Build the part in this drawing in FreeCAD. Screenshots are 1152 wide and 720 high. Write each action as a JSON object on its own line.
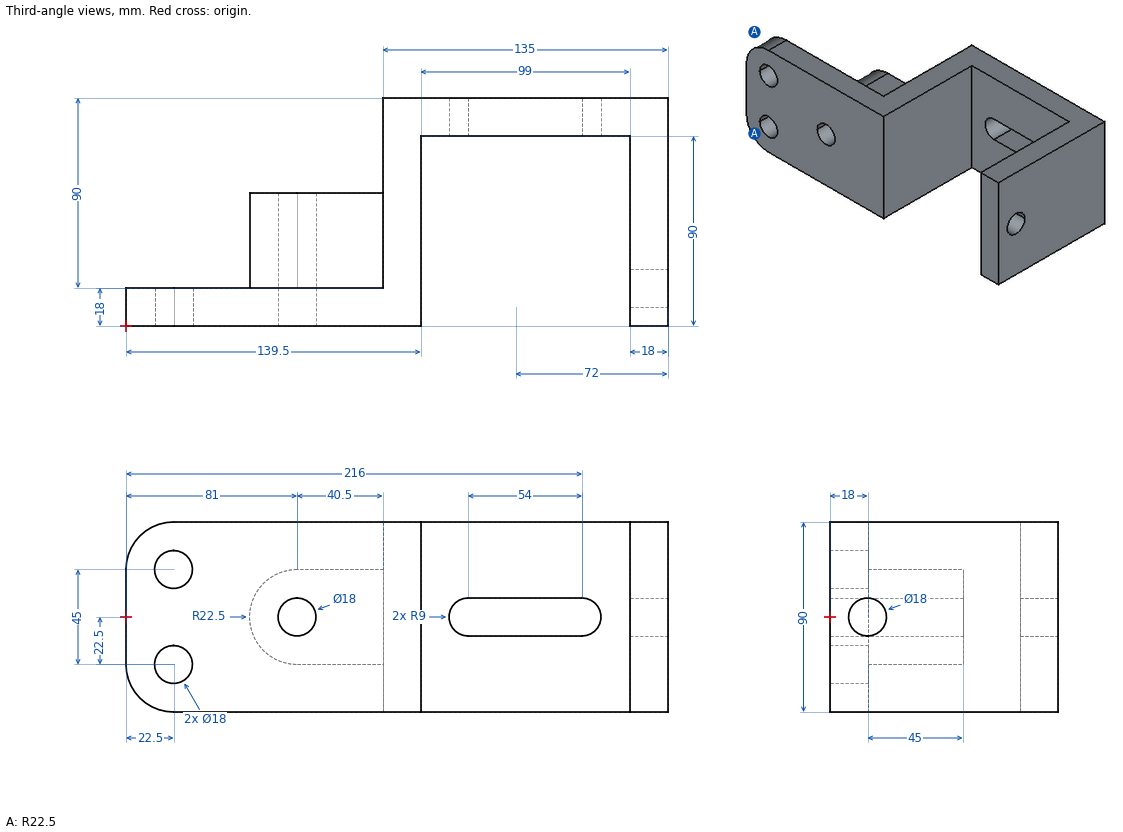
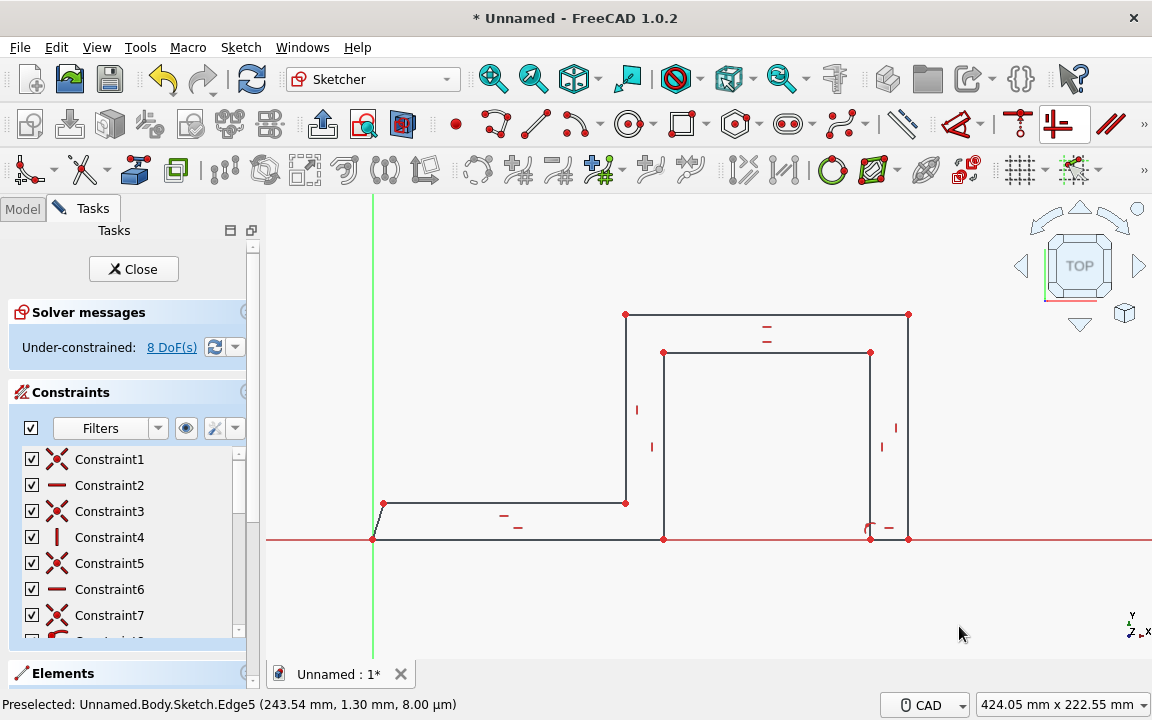
{"action": "scroll", "coordinate": [381, 514], "scroll_direction": "up", "scroll_amount": 3}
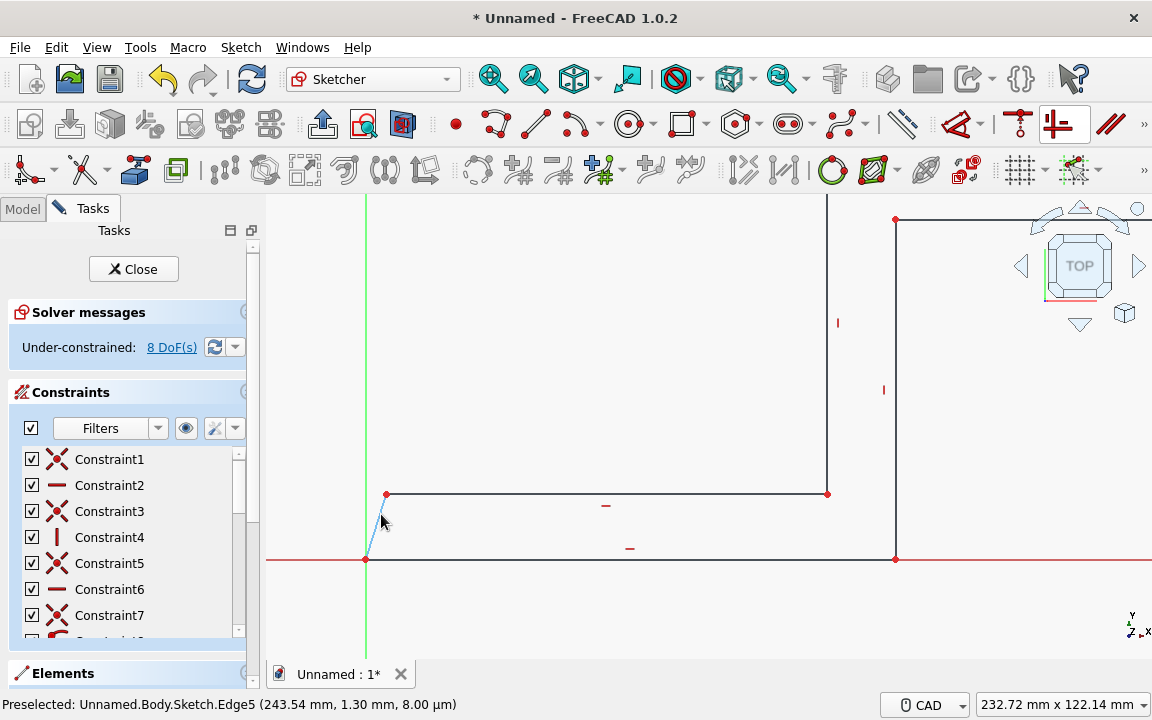
{"action": "left_click", "coordinate": [380, 514]}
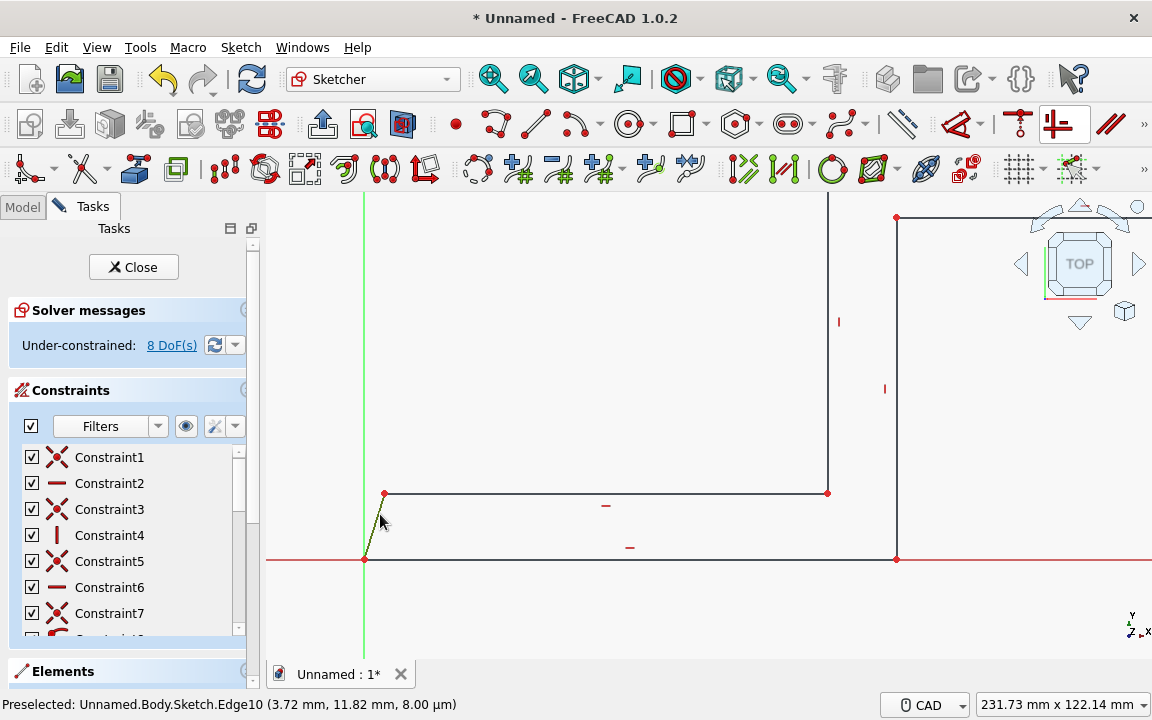
{"action": "left_click", "coordinate": [1084, 124]}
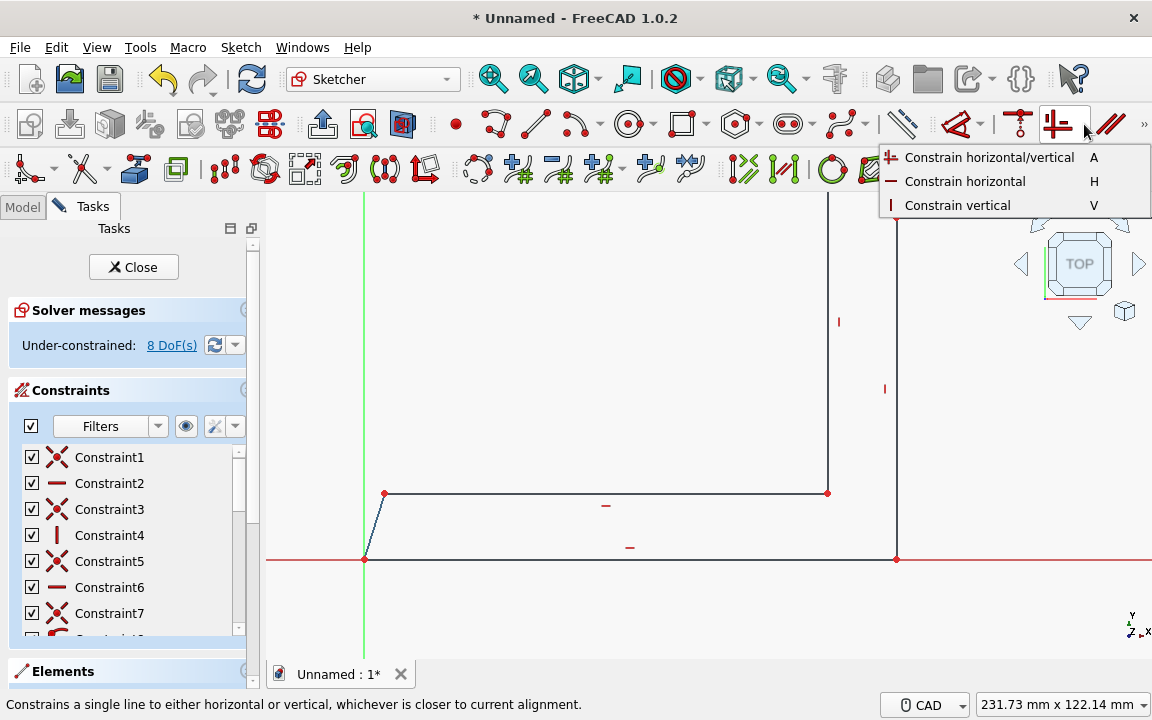
{"action": "left_click", "coordinate": [1015, 205]}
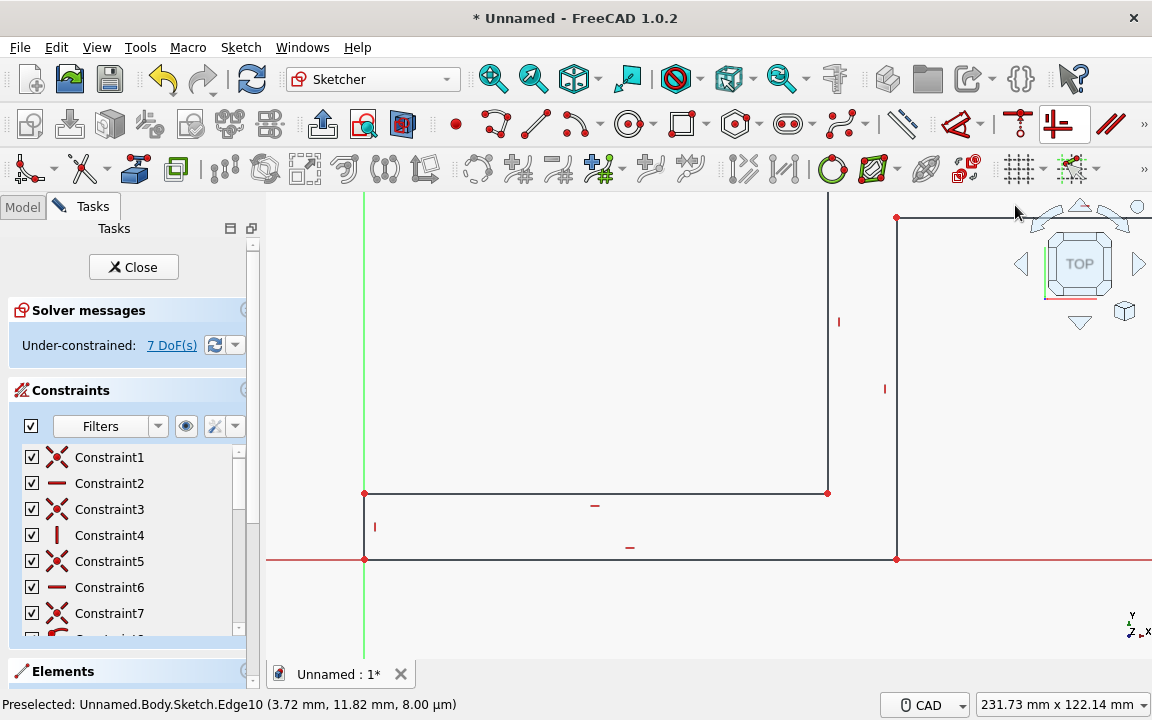
{"action": "left_click", "coordinate": [956, 124]}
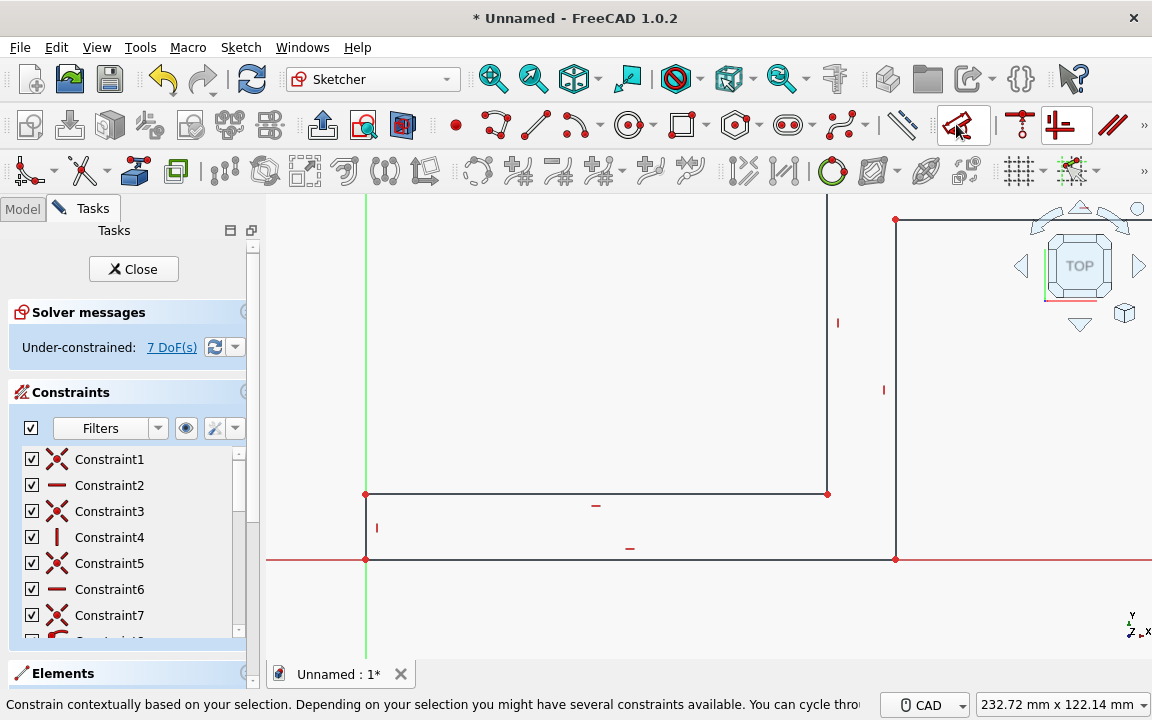
{"action": "left_click", "coordinate": [896, 458]}
{"action": "left_click", "coordinate": [930, 391]}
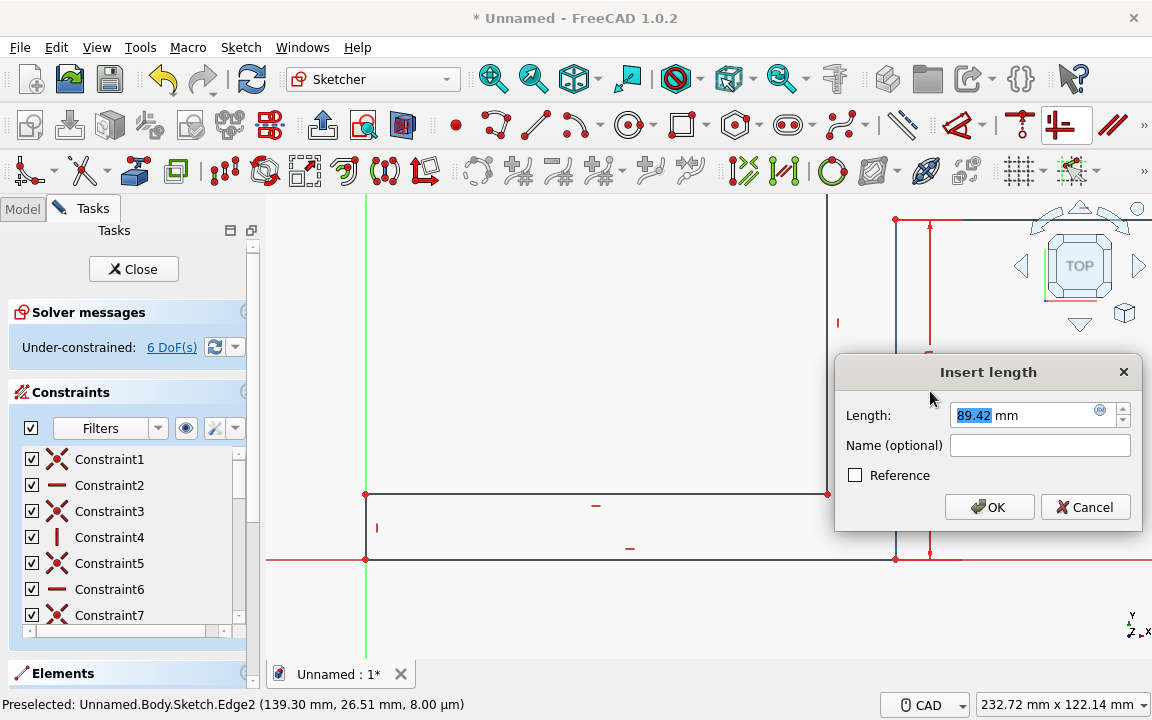
{"action": "type", "text": "90"}
{"action": "key", "text": "Return"}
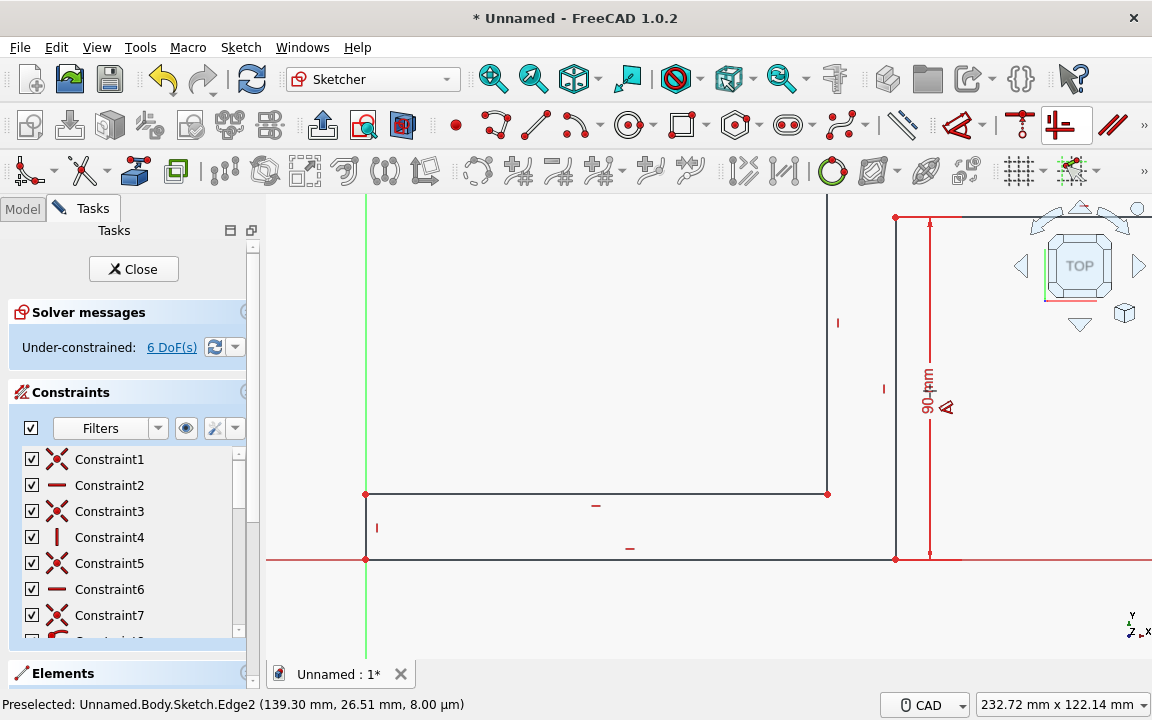
{"action": "scroll", "coordinate": [381, 514], "scroll_direction": "down", "scroll_amount": 3}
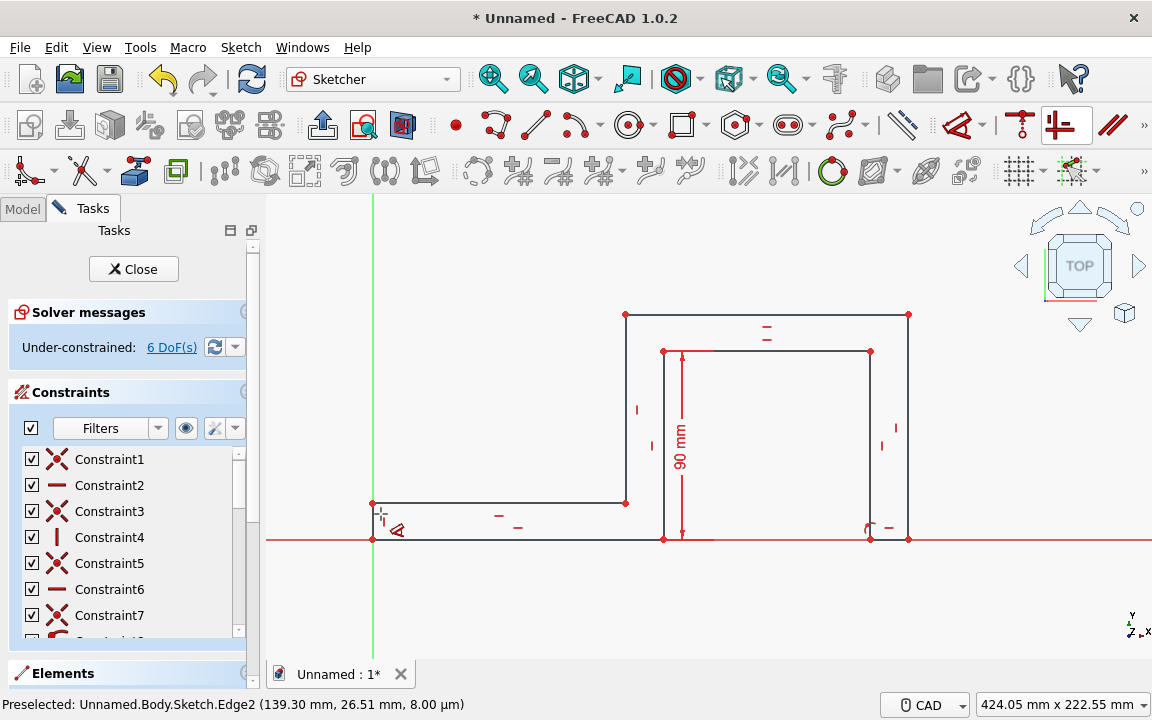
{"action": "left_click", "coordinate": [726, 351]}
{"action": "left_click", "coordinate": [767, 385]}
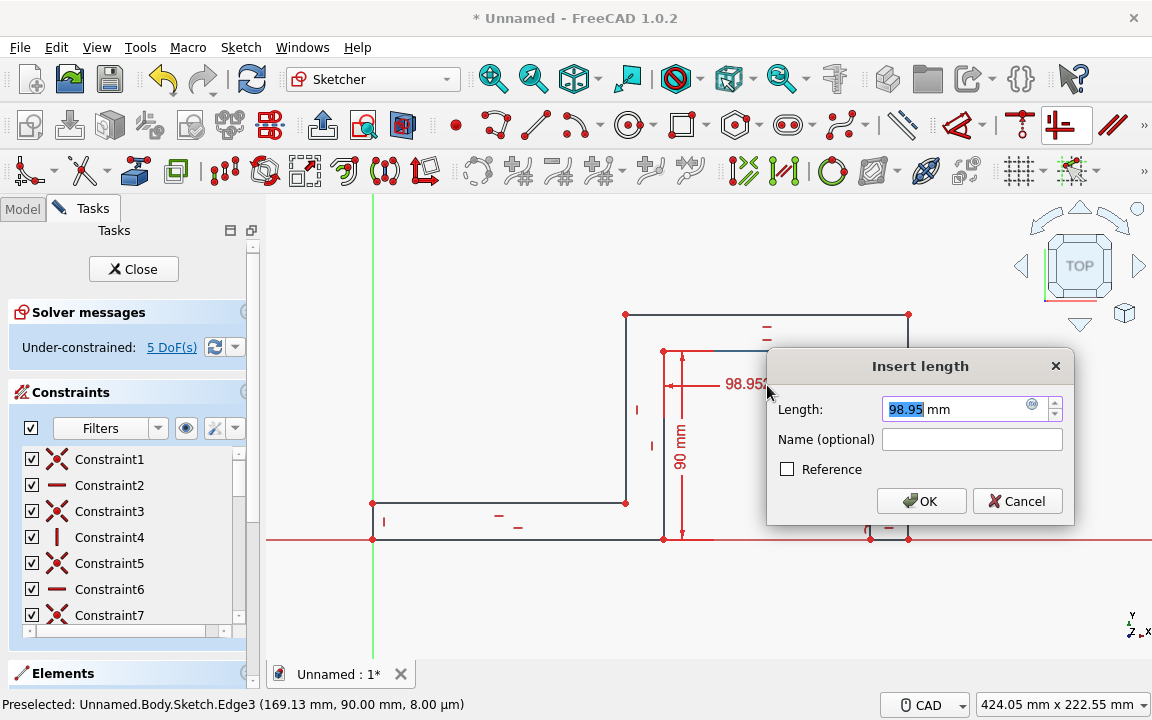
{"action": "type", "text": "99"}
{"action": "key", "text": "Return"}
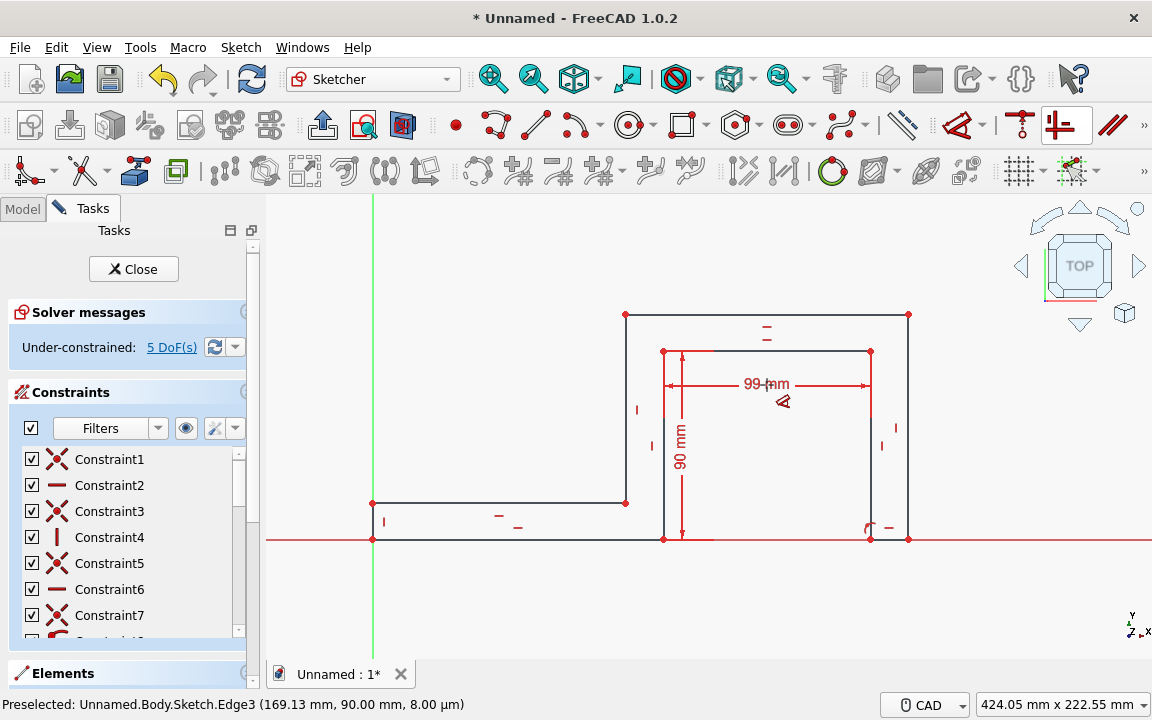
{"action": "scroll", "coordinate": [882, 540], "scroll_direction": "up", "scroll_amount": 2}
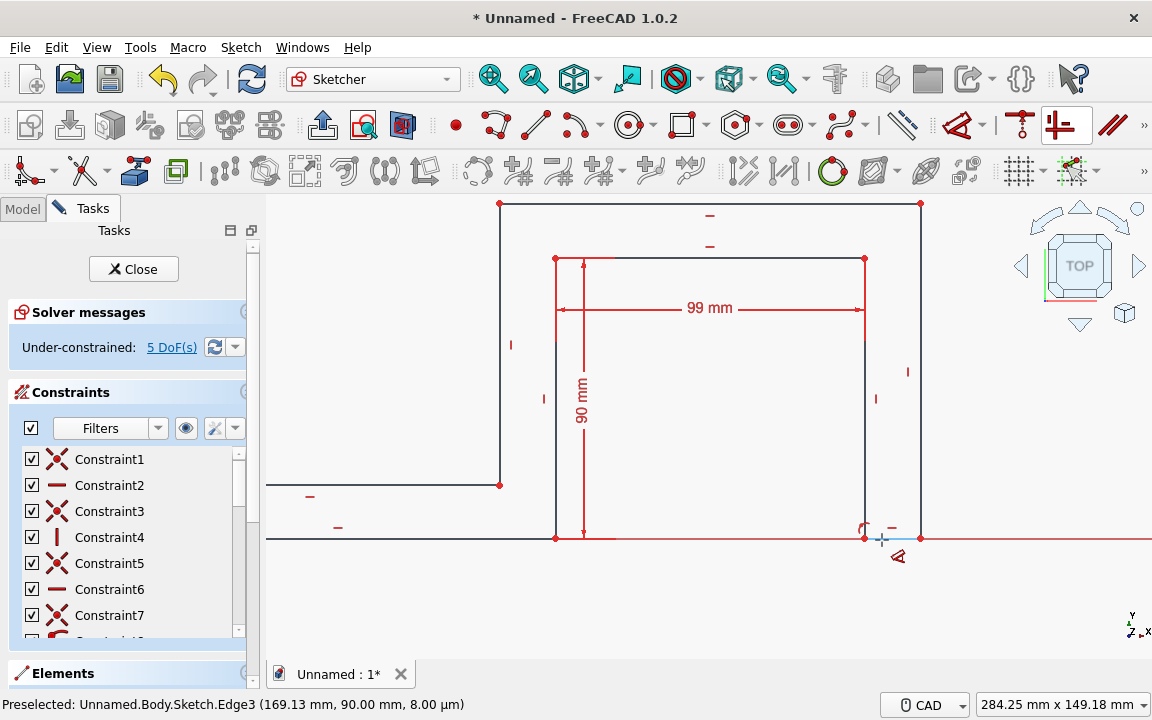
{"action": "left_click", "coordinate": [881, 539]}
{"action": "left_click", "coordinate": [893, 573]}